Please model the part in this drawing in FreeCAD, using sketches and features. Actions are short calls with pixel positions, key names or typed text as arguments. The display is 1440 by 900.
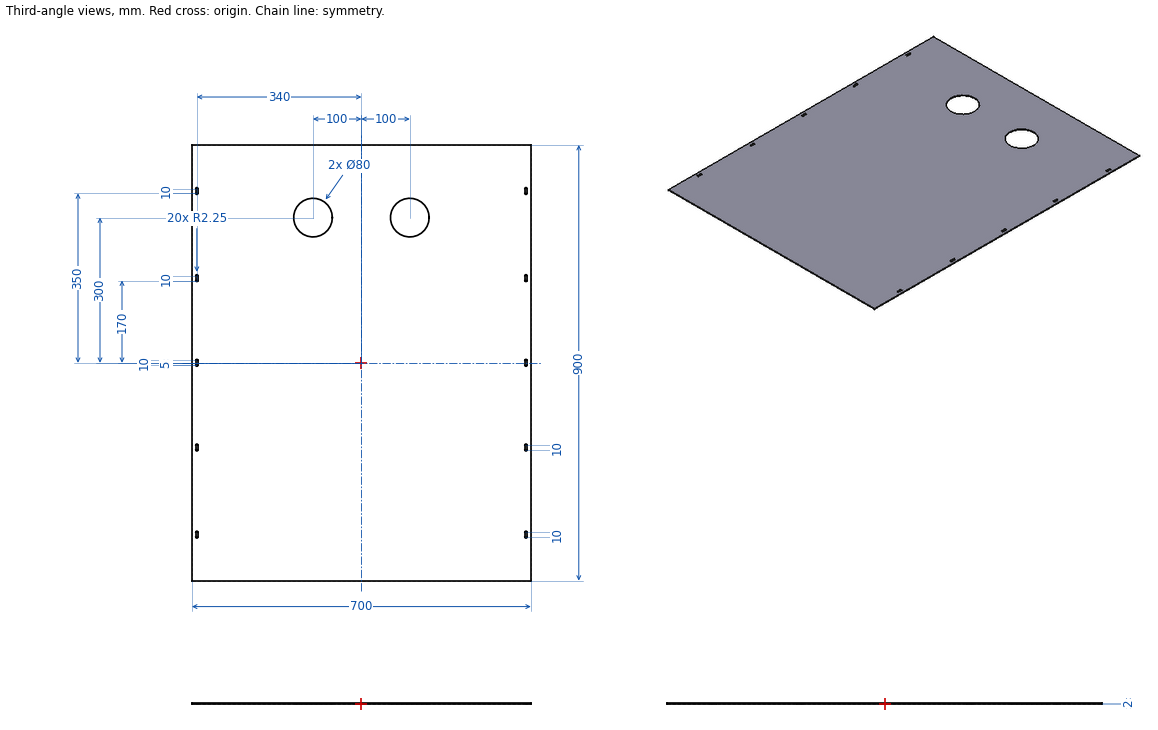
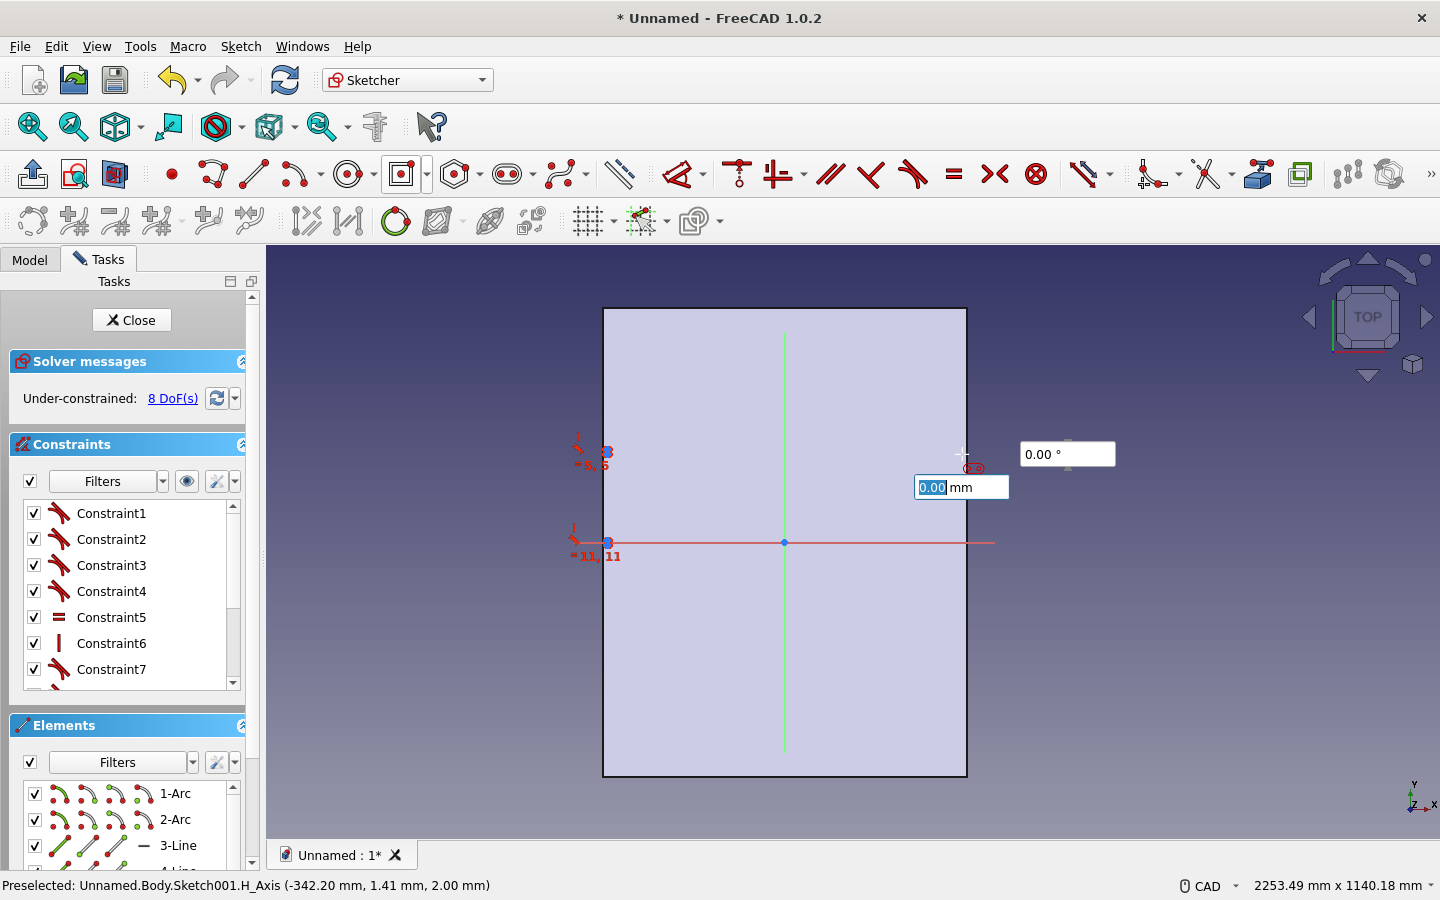
scroll(962, 449, up, 6)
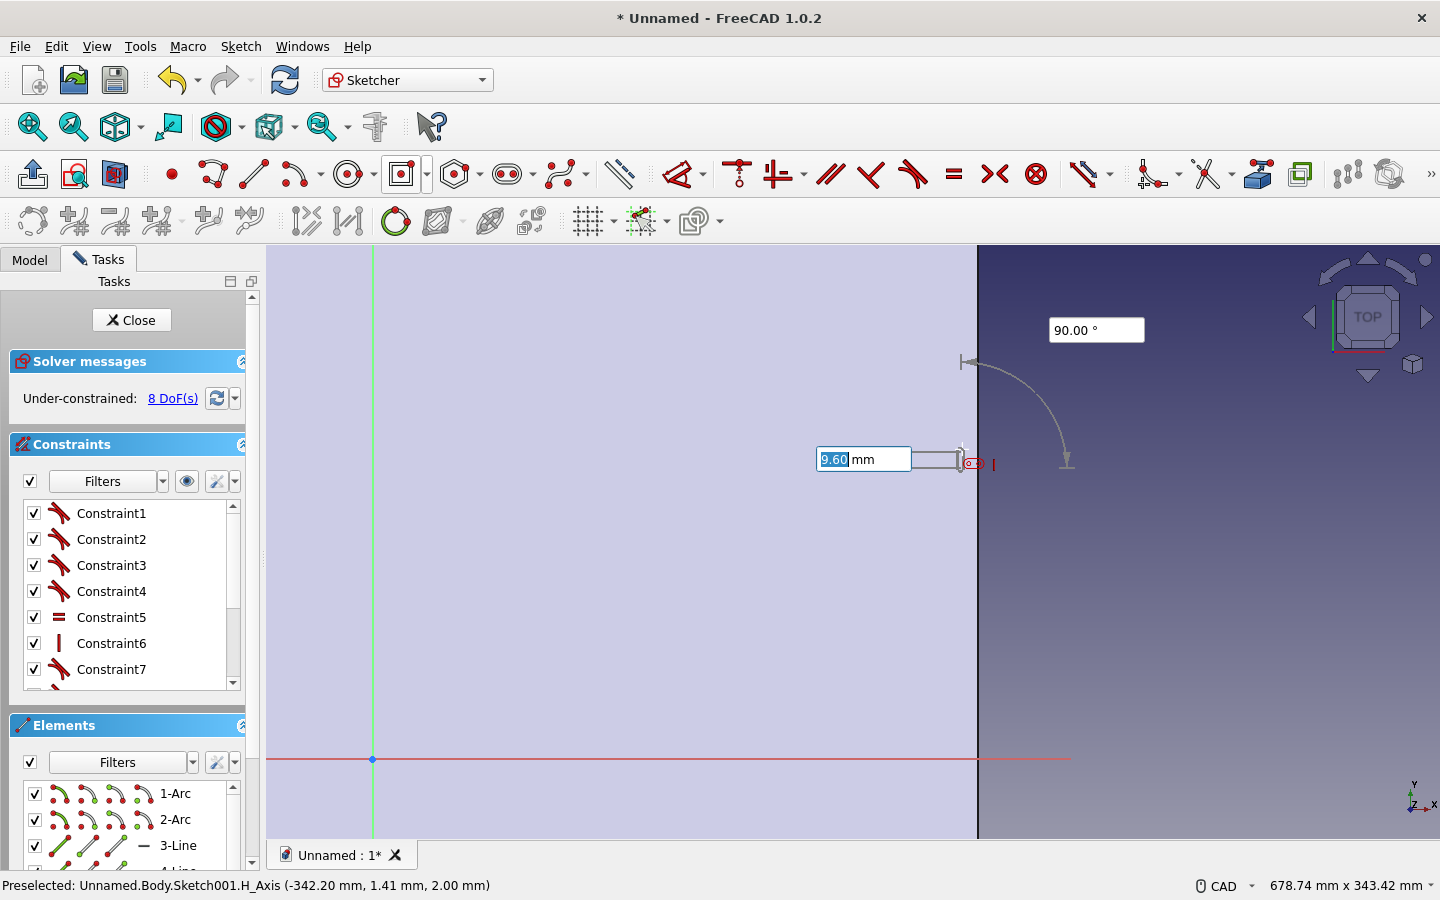
click(961, 448)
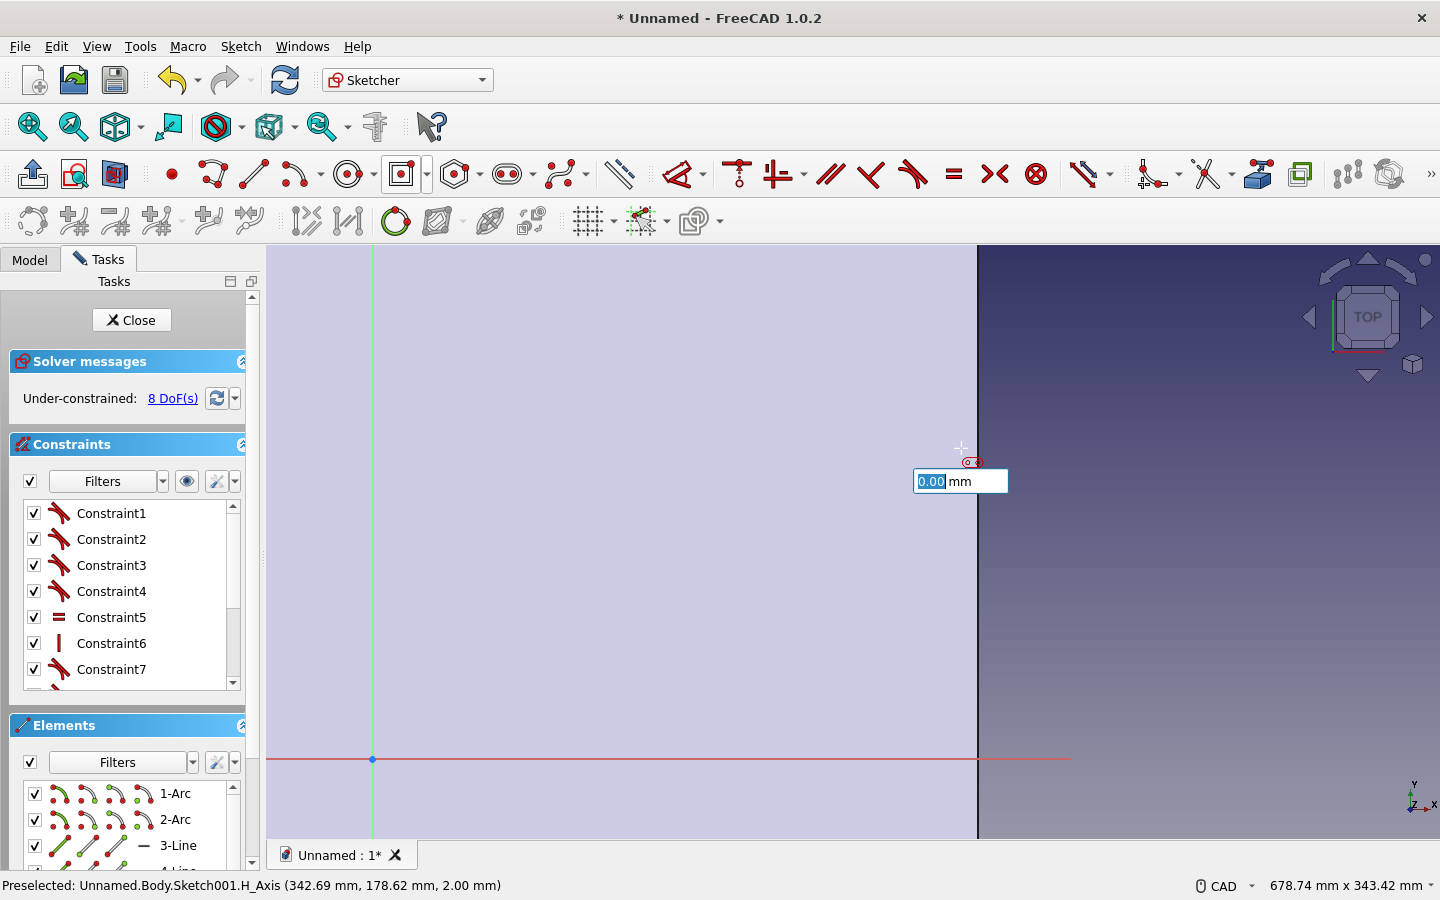
scroll(957, 456, up, 8)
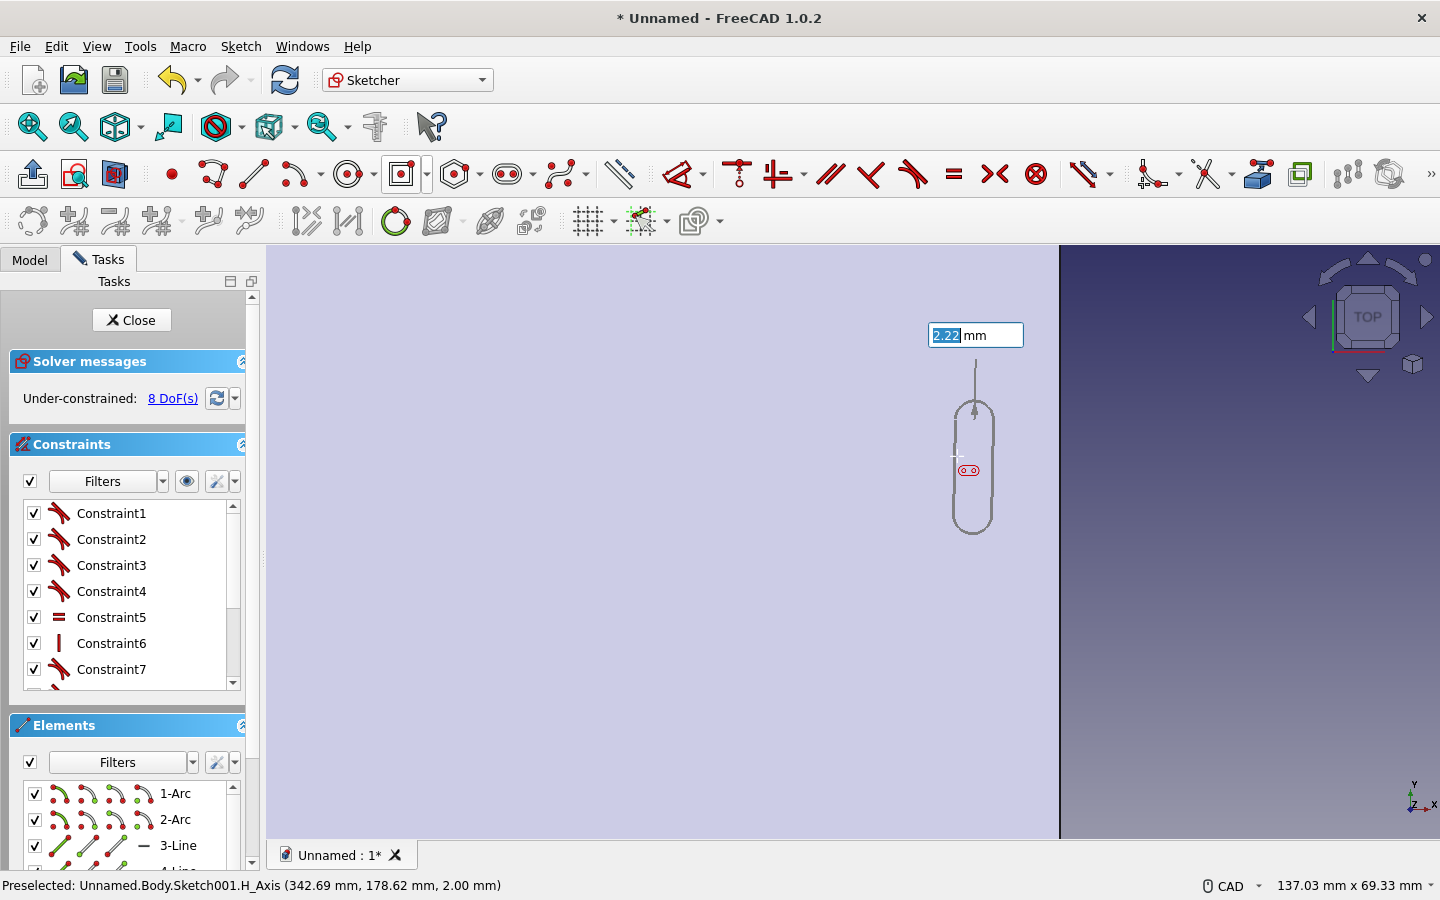
click(955, 456)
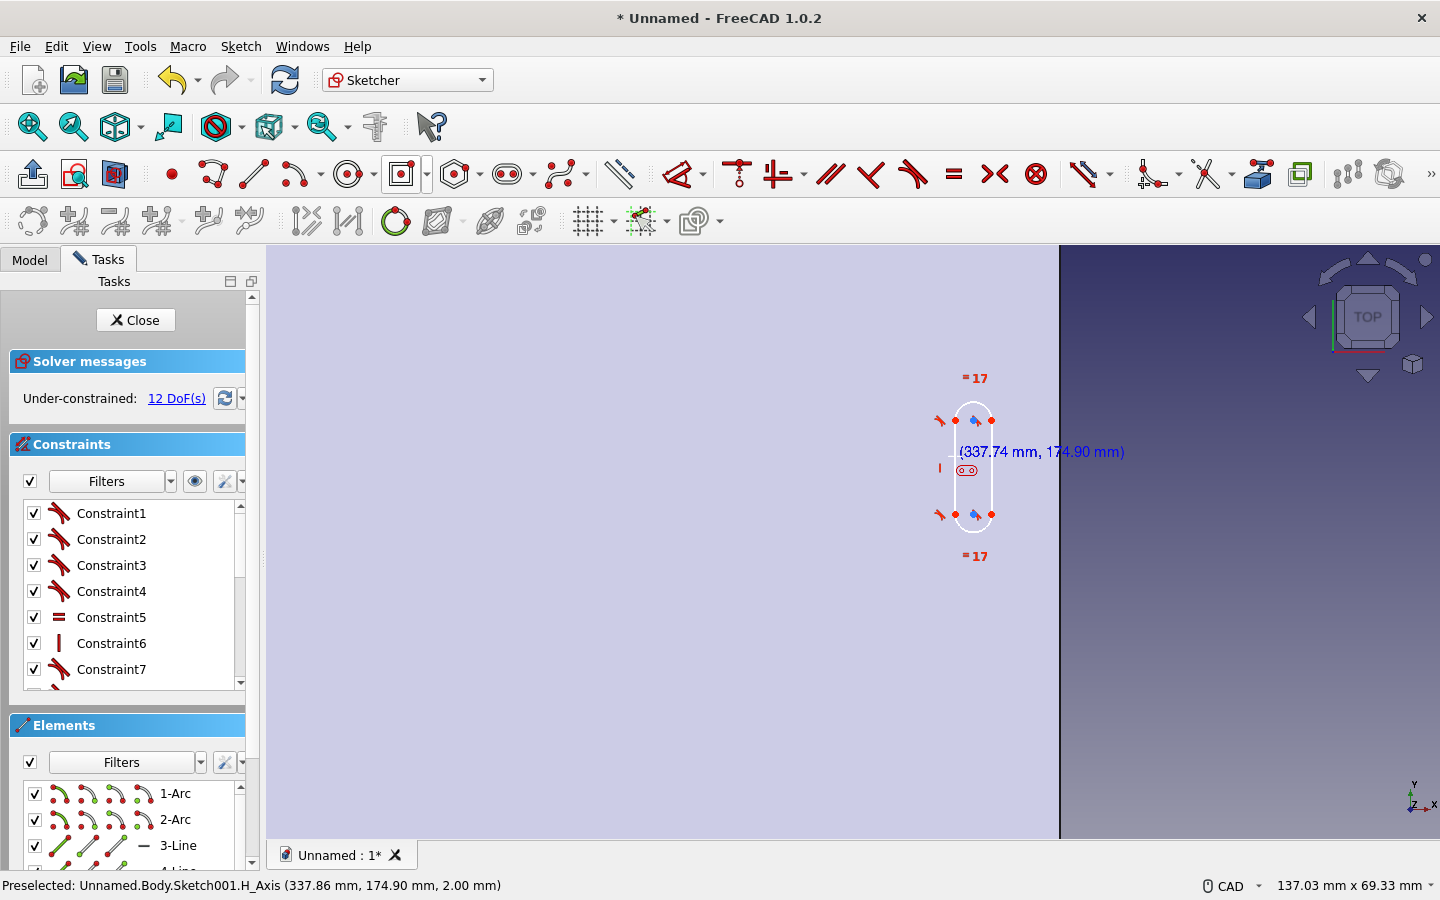
scroll(961, 450, down, 14)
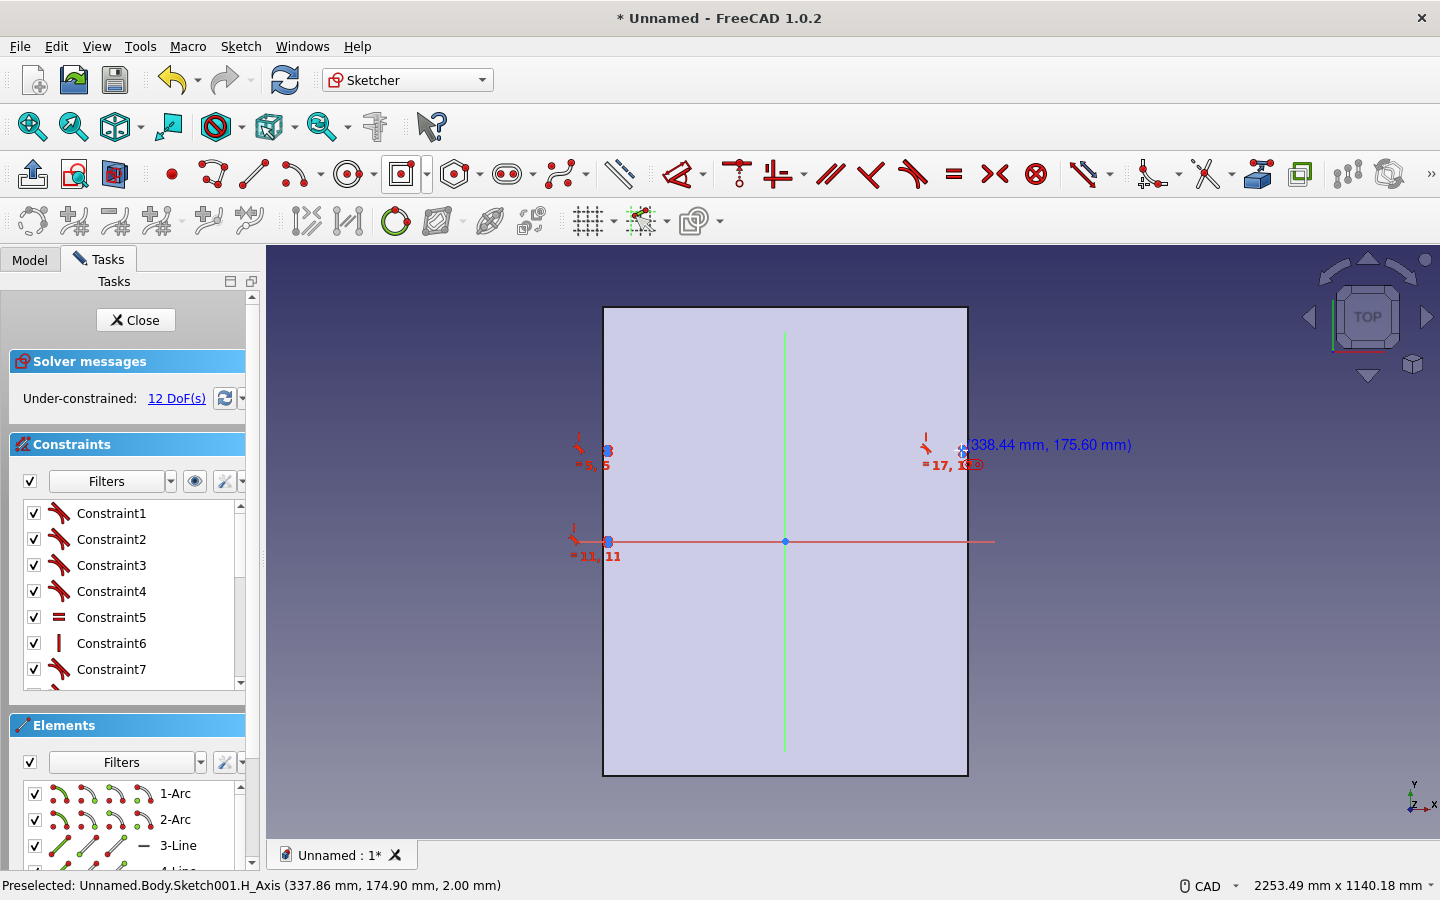
scroll(962, 544, up, 15)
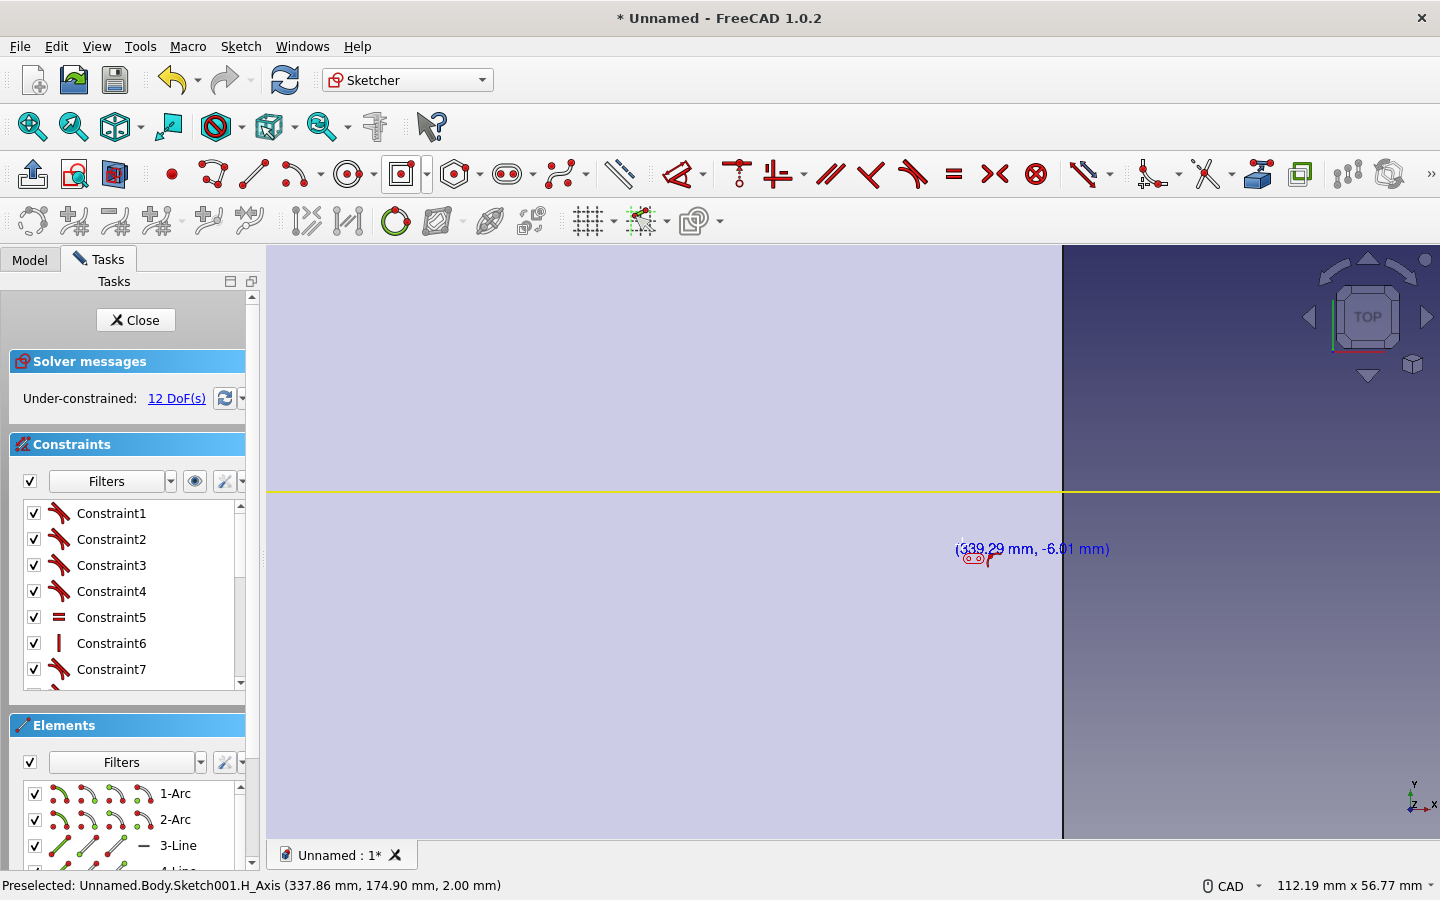
scroll(962, 545, down, 15)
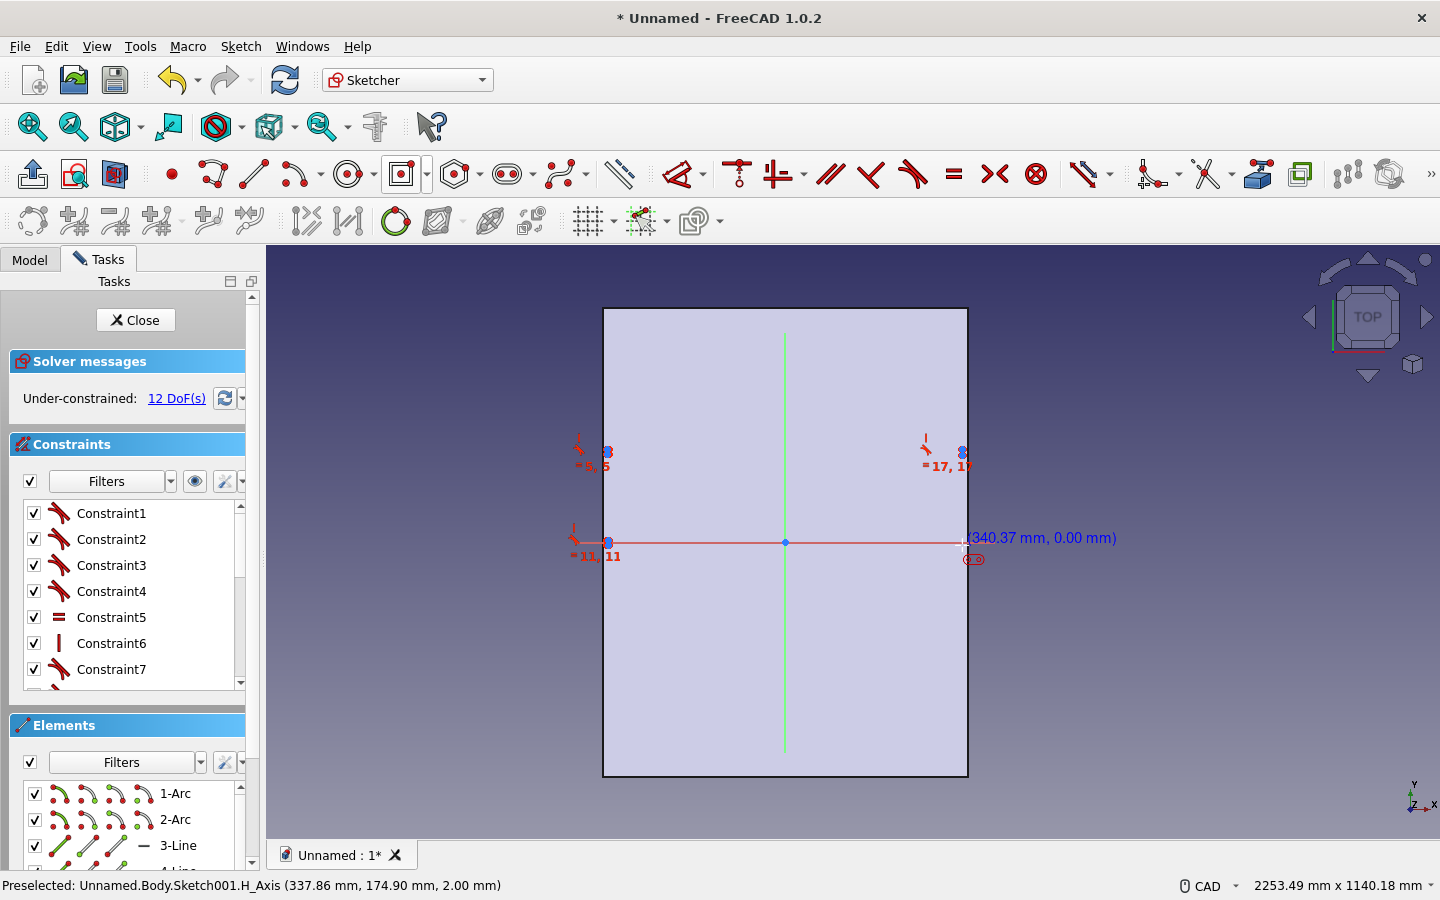
scroll(962, 545, up, 10)